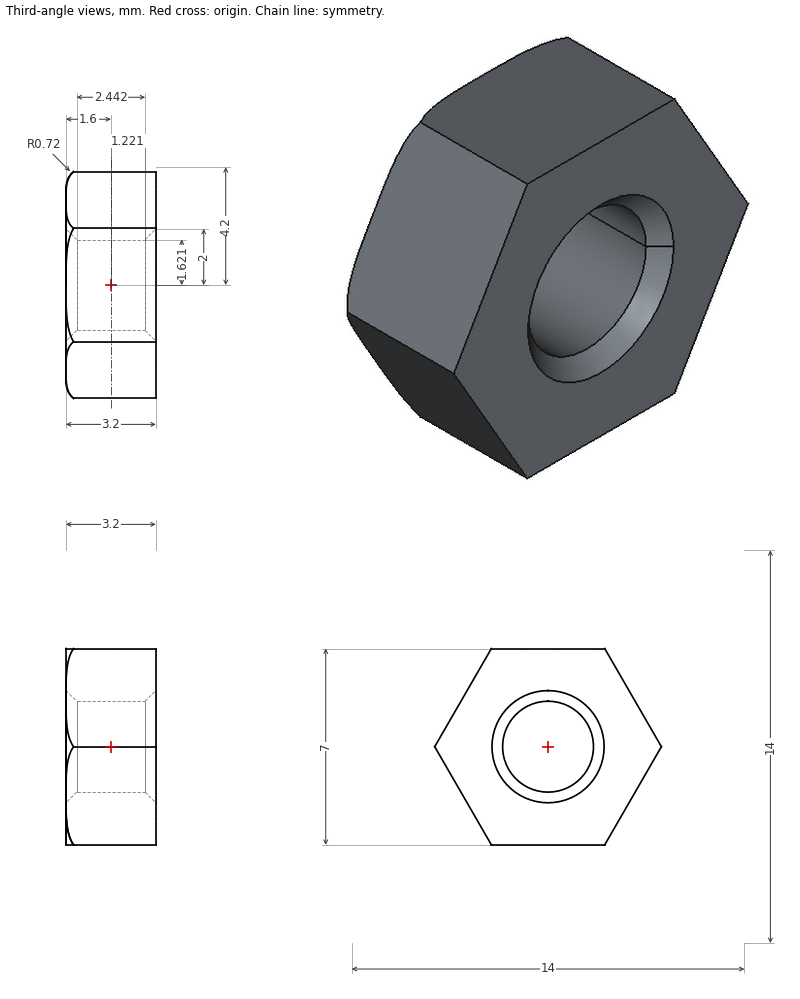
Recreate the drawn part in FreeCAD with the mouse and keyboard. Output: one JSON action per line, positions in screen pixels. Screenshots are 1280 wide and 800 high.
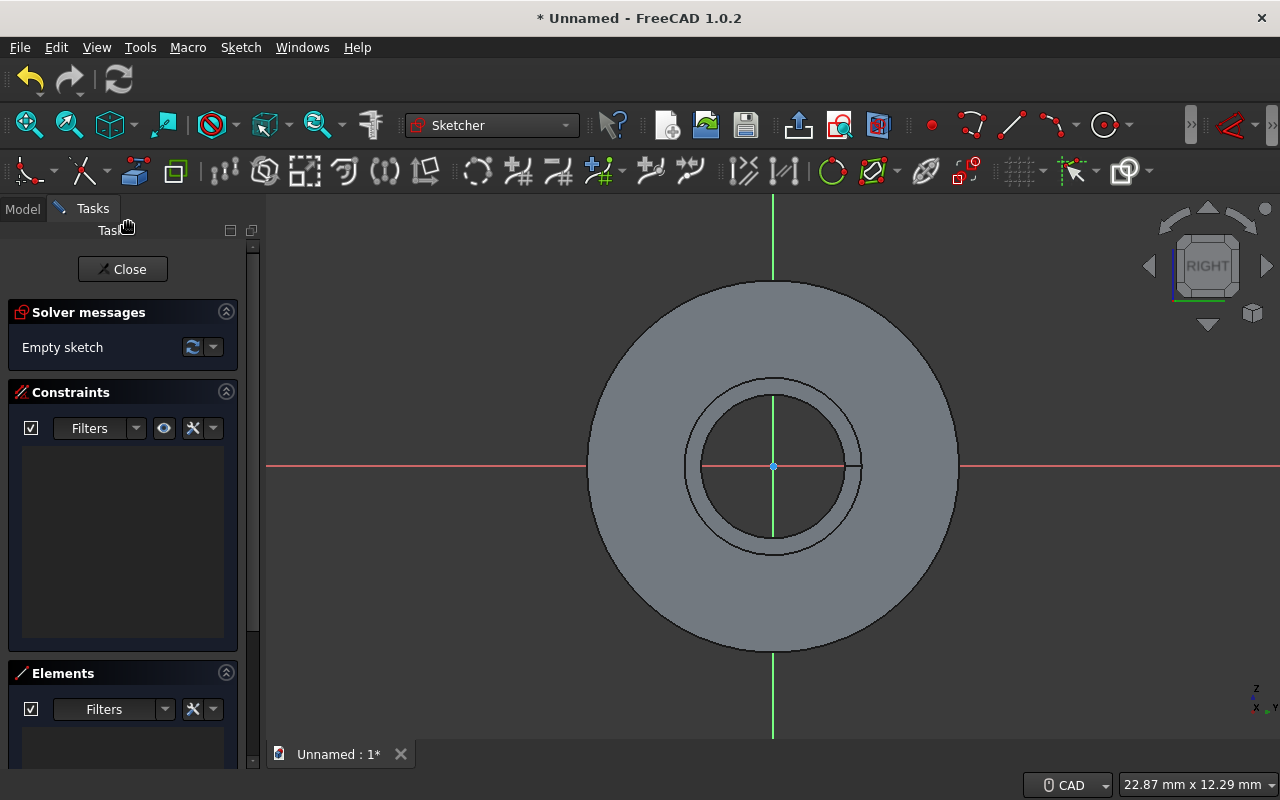
{"action": "key", "text": "q s"}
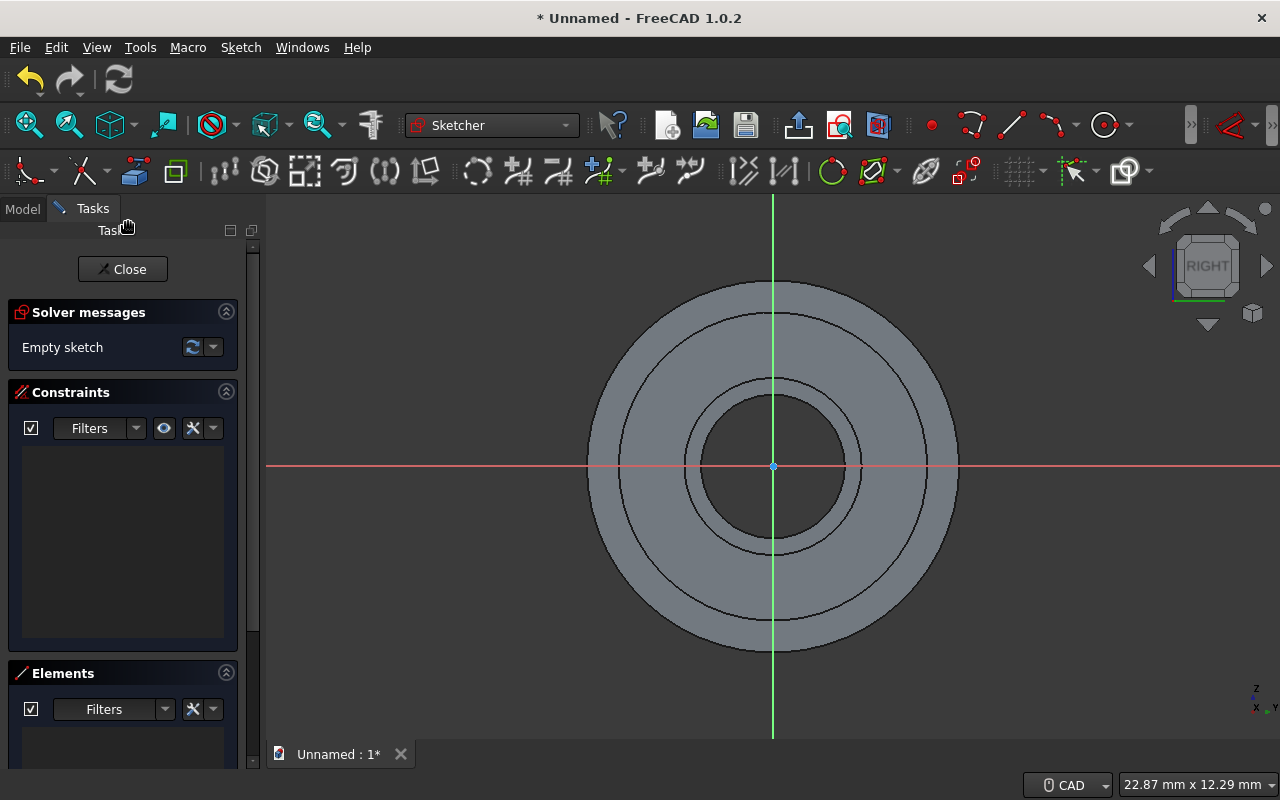
{"action": "scroll", "coordinate": [621, 467], "scroll_direction": "down", "scroll_amount": 3}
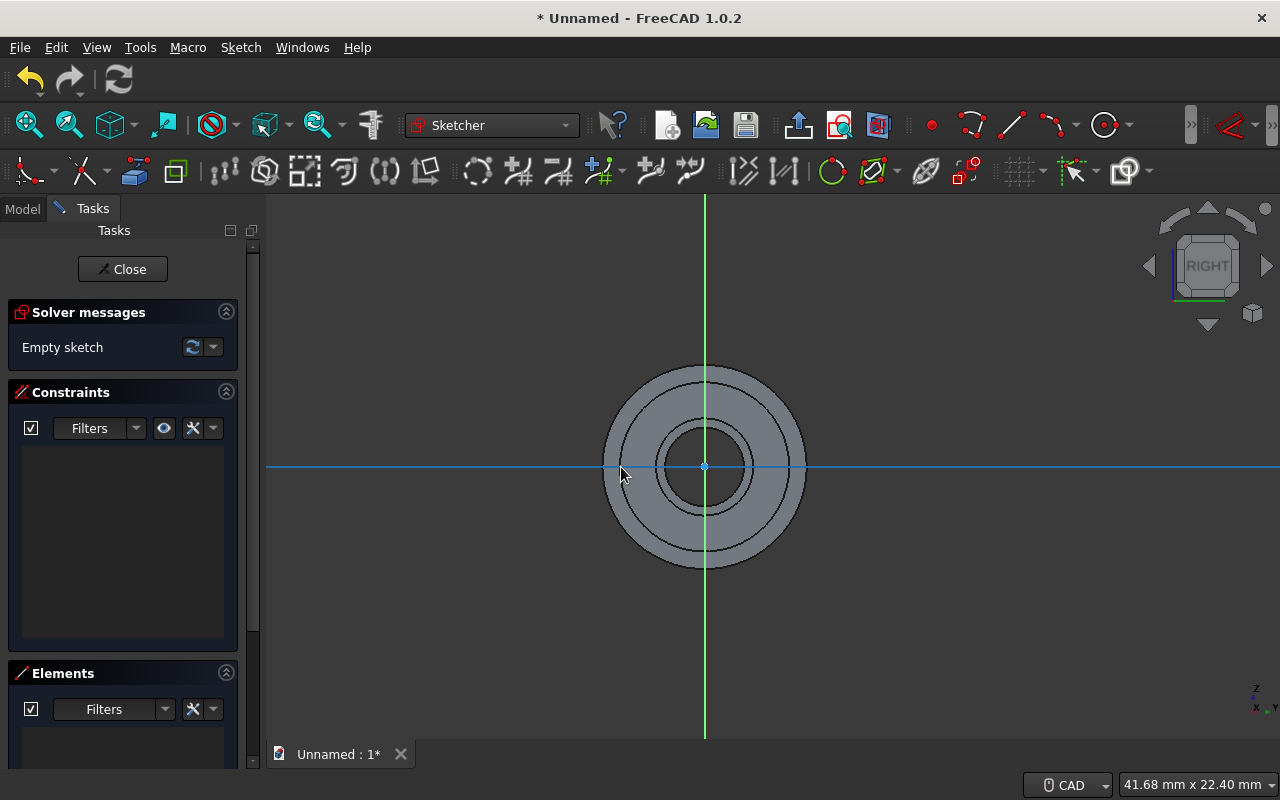
{"action": "key", "text": "g v"}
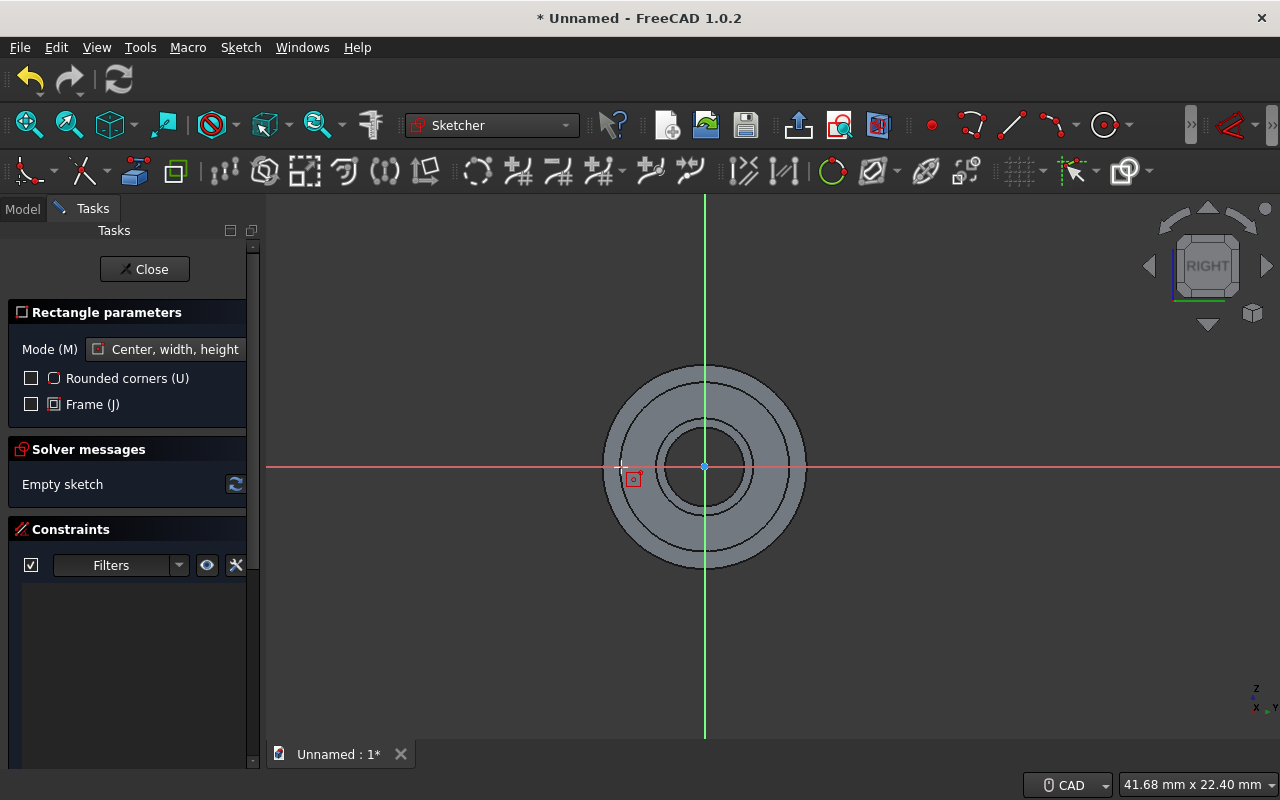
{"action": "left_click", "coordinate": [705, 467]}
{"action": "mouse_move", "coordinate": [875, 297]}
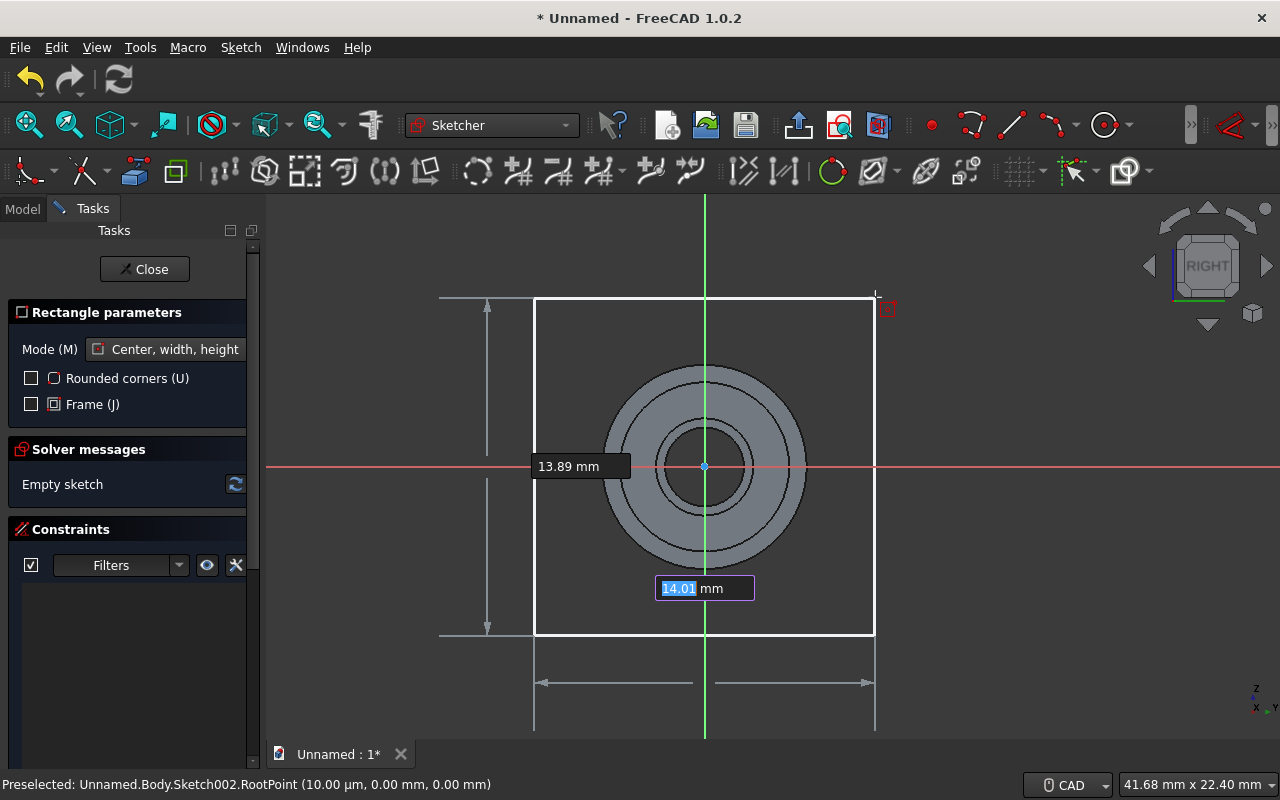
{"action": "type", "text": "14"}
{"action": "key", "text": "Tab"}
{"action": "type", "text": "14"}
{"action": "key", "text": "Return"}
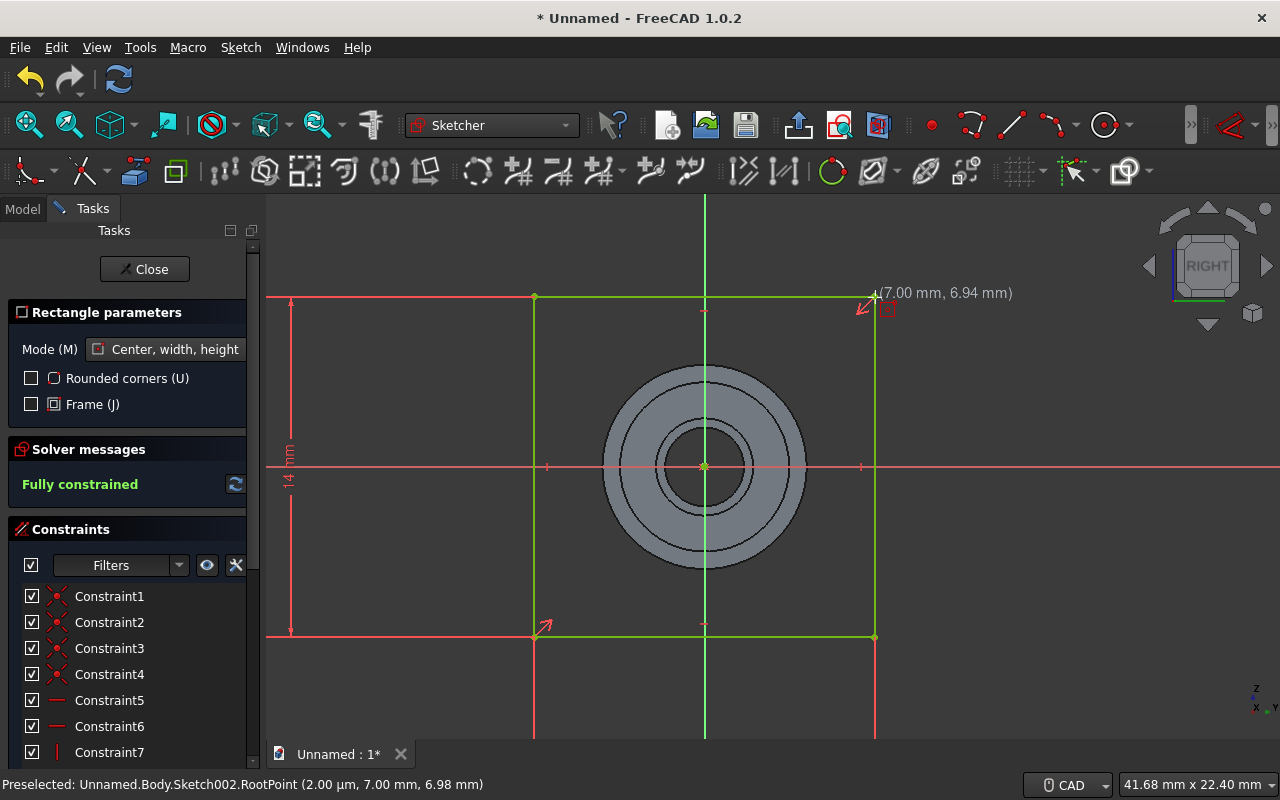
{"action": "key", "text": "g p 6"}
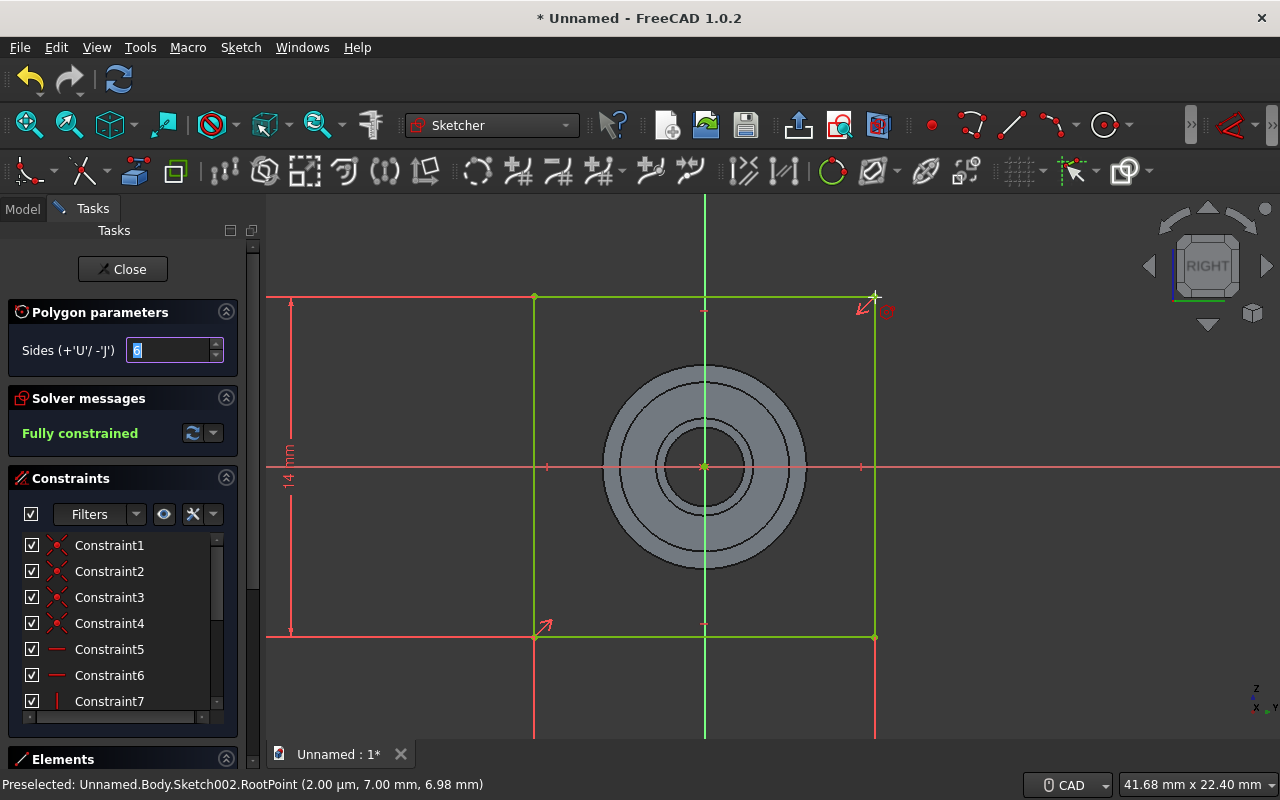
{"action": "left_click", "coordinate": [705, 467]}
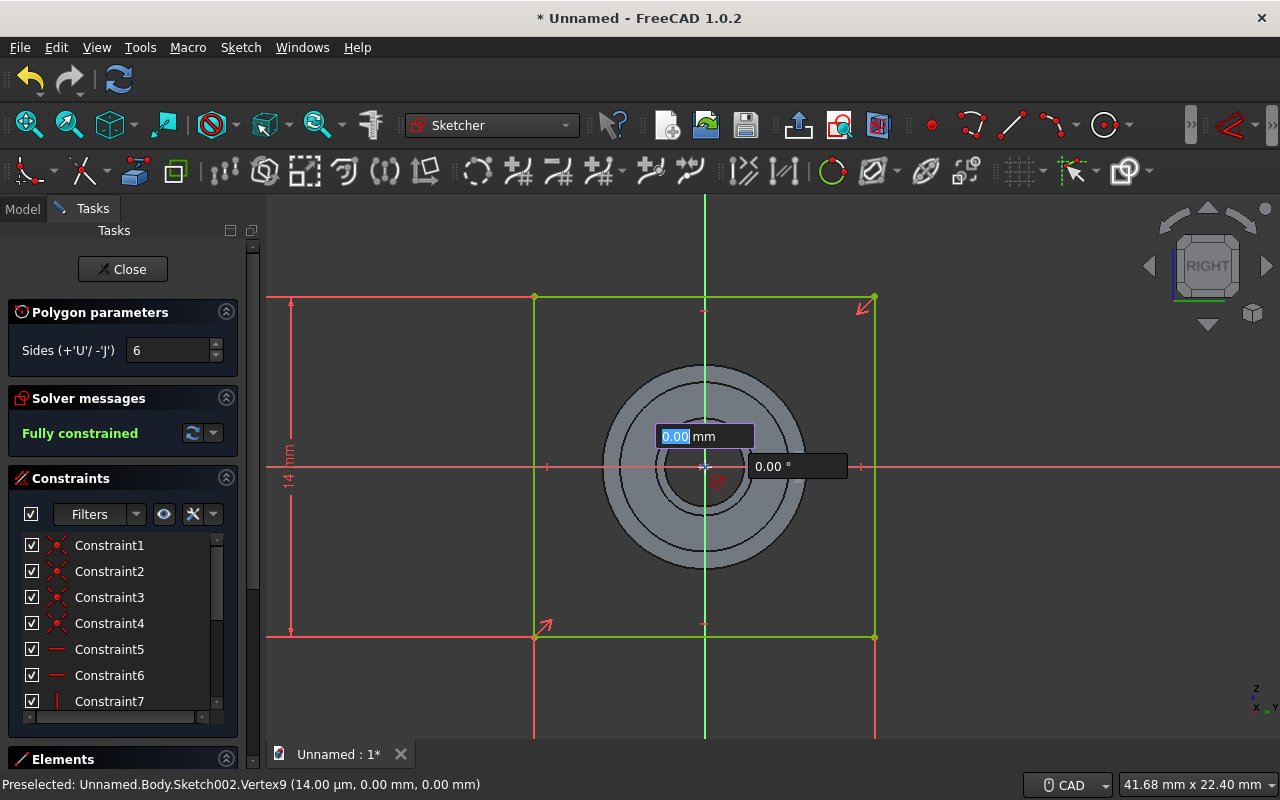
{"action": "left_click", "coordinate": [803, 467]}
{"action": "right_click", "coordinate": [803, 467]}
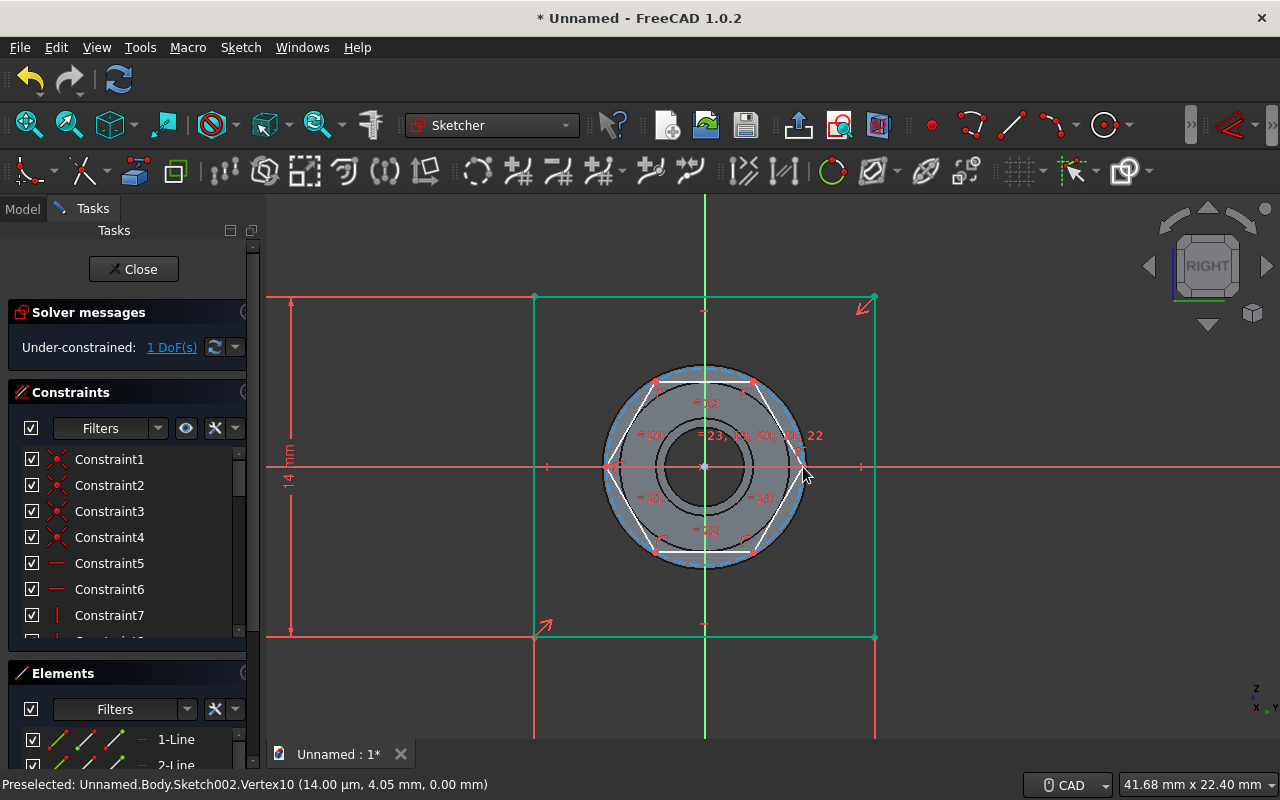
{"action": "left_click", "coordinate": [1230, 126]}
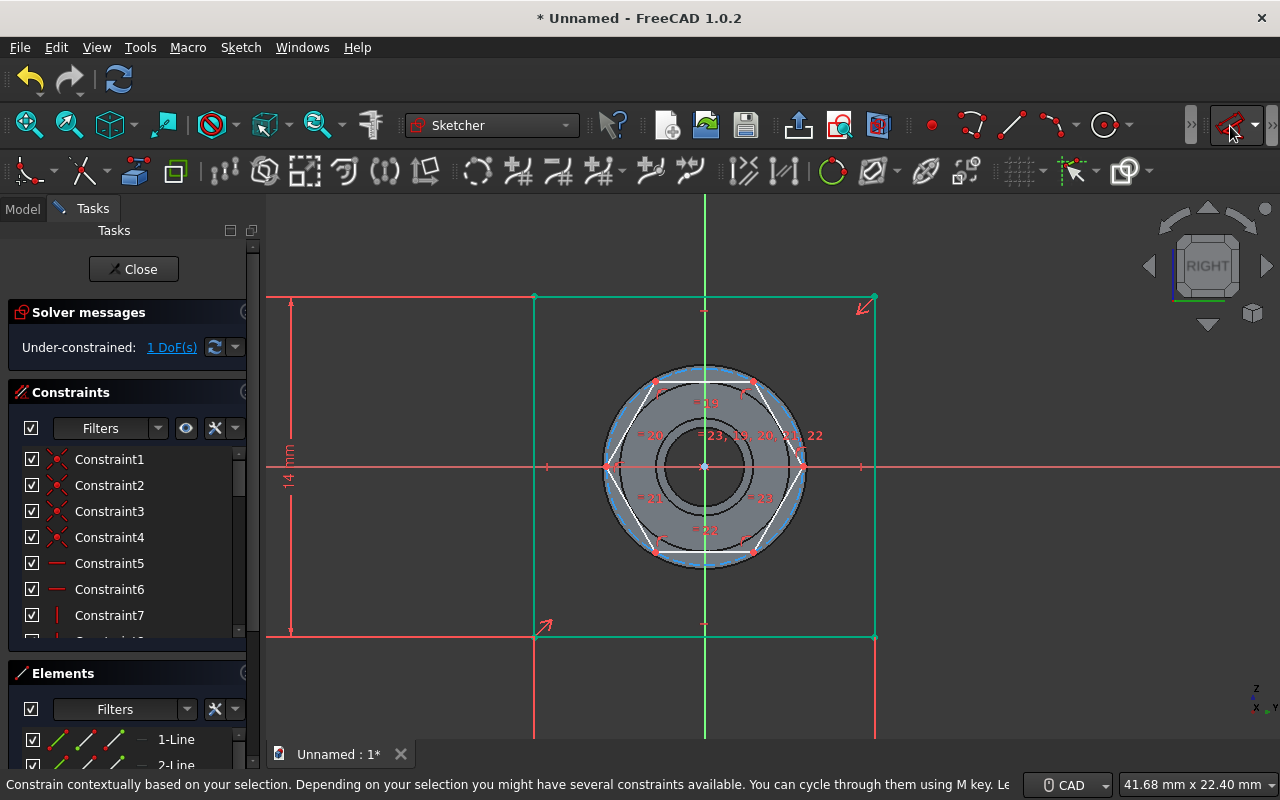
{"action": "left_click", "coordinate": [655, 552]}